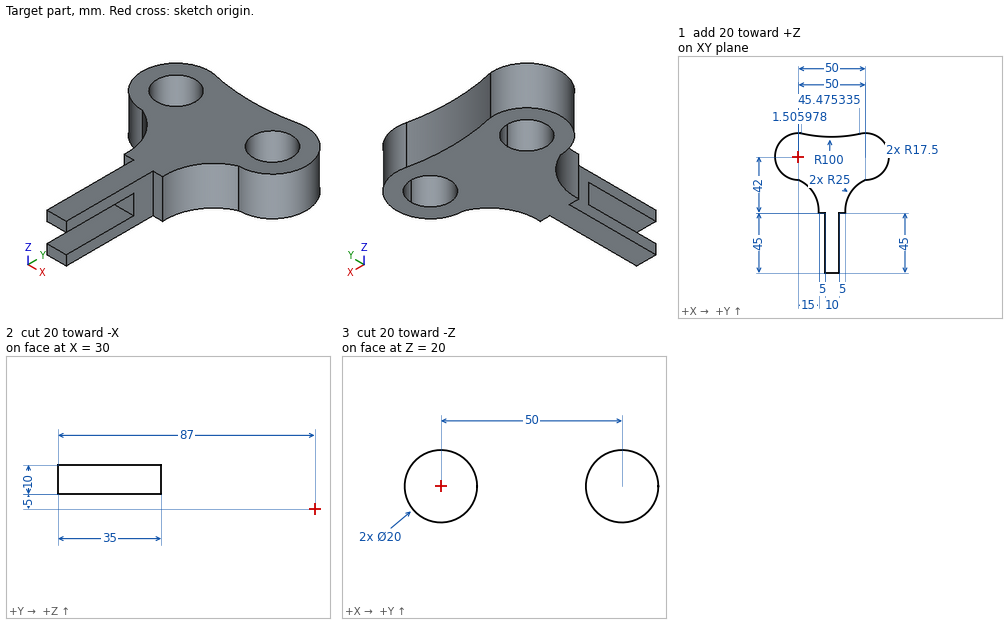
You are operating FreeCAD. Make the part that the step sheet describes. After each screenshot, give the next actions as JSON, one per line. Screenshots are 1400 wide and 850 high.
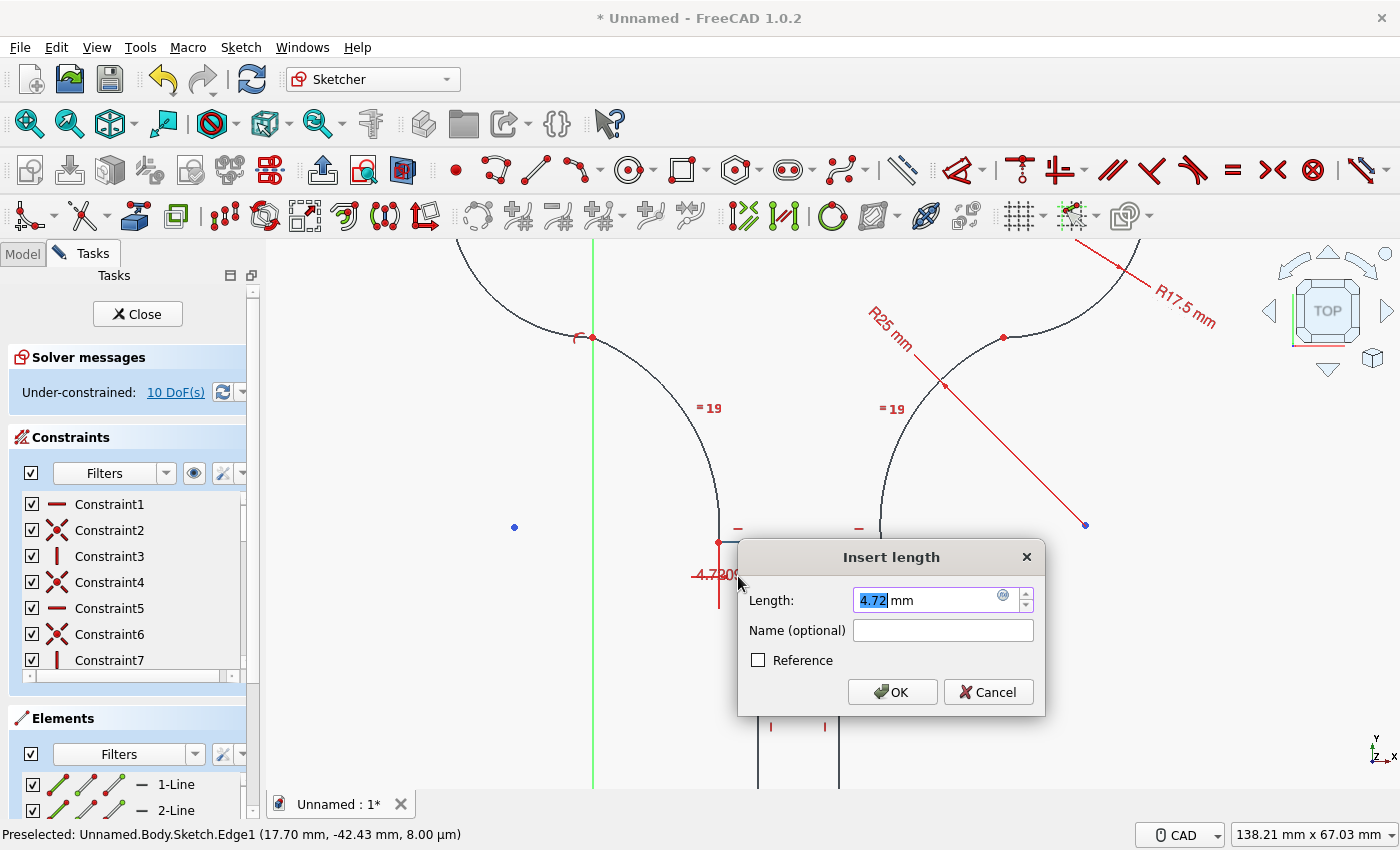
{"action": "type", "text": "5"}
{"action": "key", "text": "Return"}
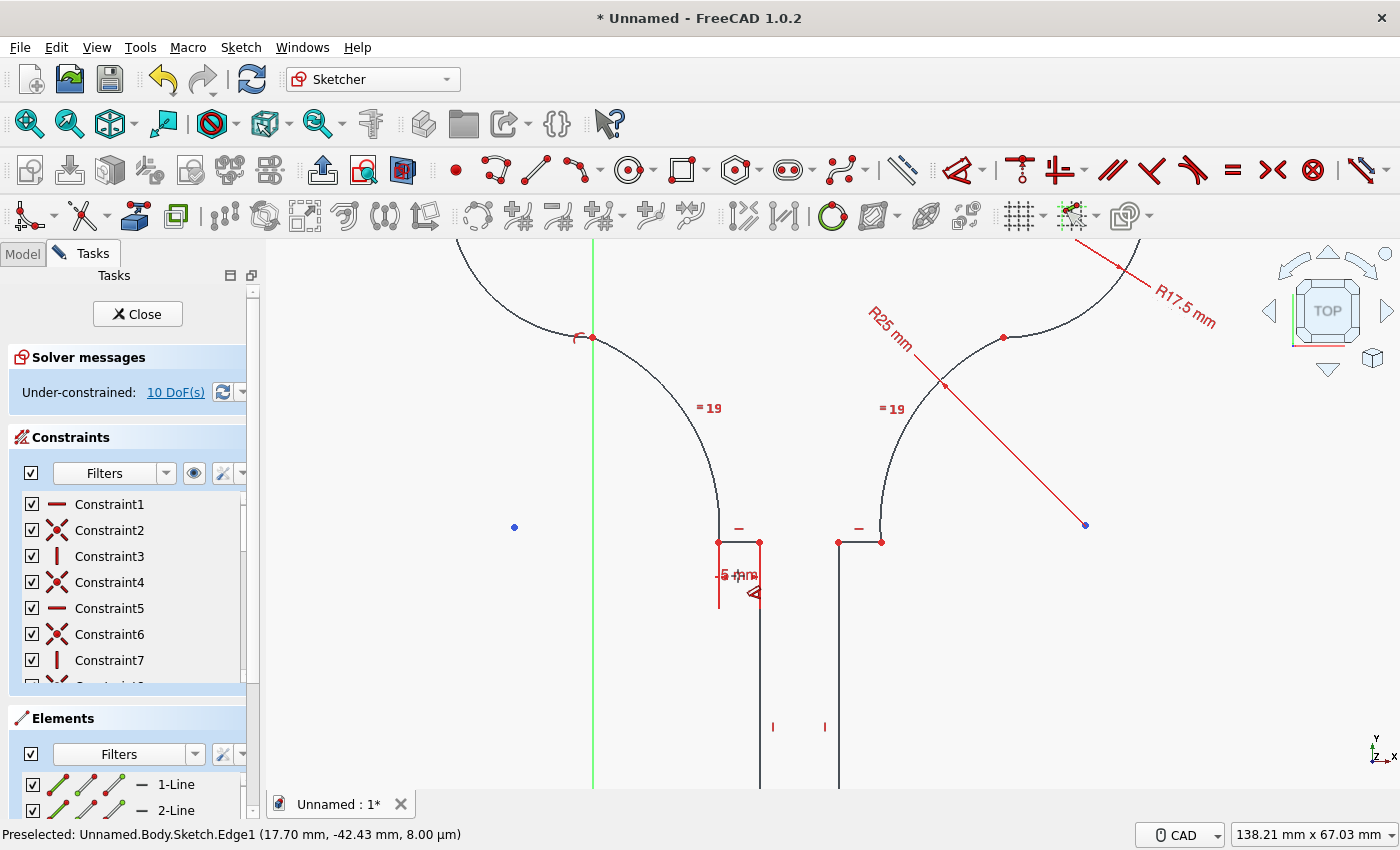
{"action": "left_click", "coordinate": [851, 542]}
{"action": "left_click", "coordinate": [860, 576]}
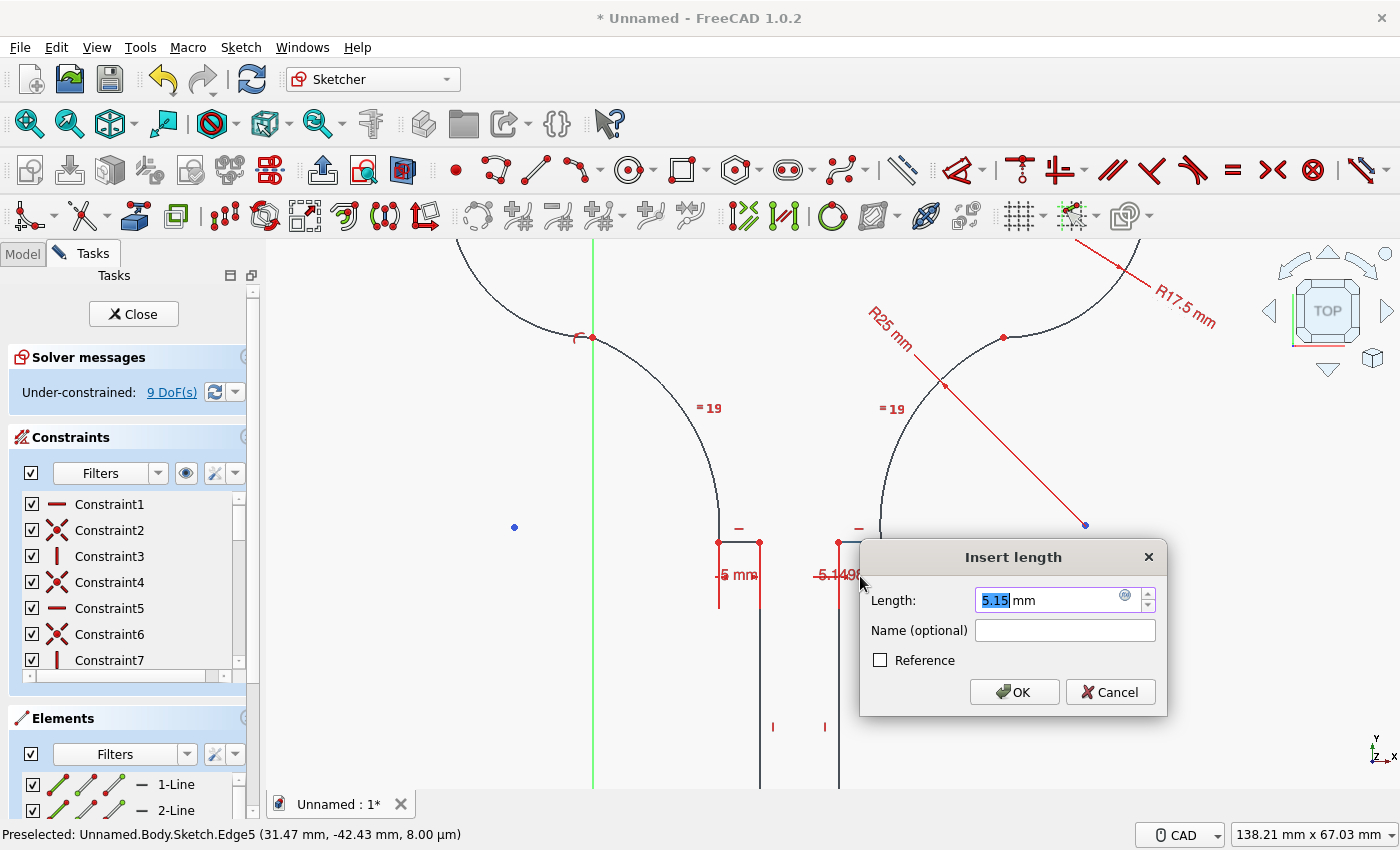
{"action": "type", "text": "5"}
{"action": "key", "text": "Return"}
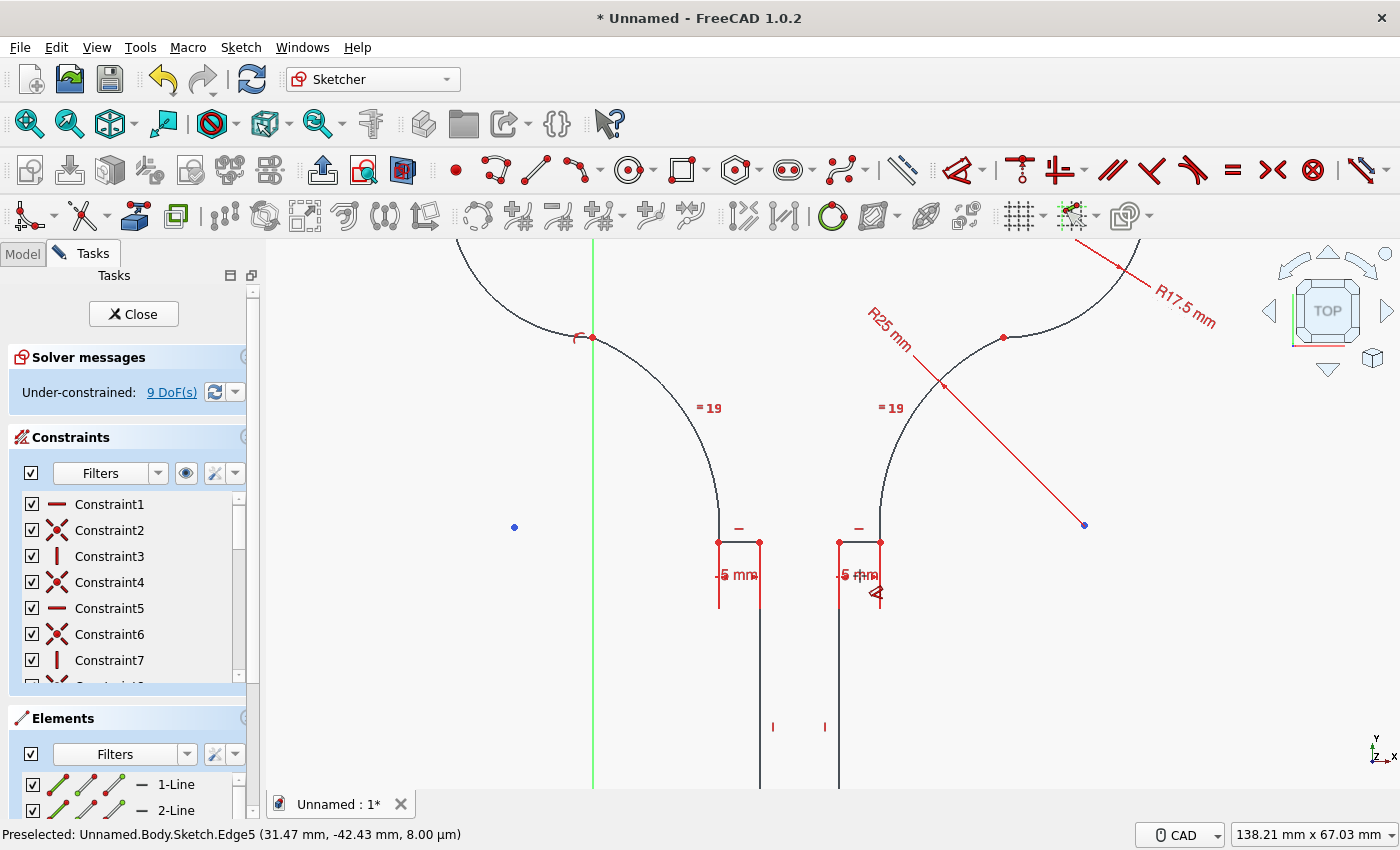
{"action": "left_click", "coordinate": [760, 653]}
{"action": "left_click", "coordinate": [726, 652]}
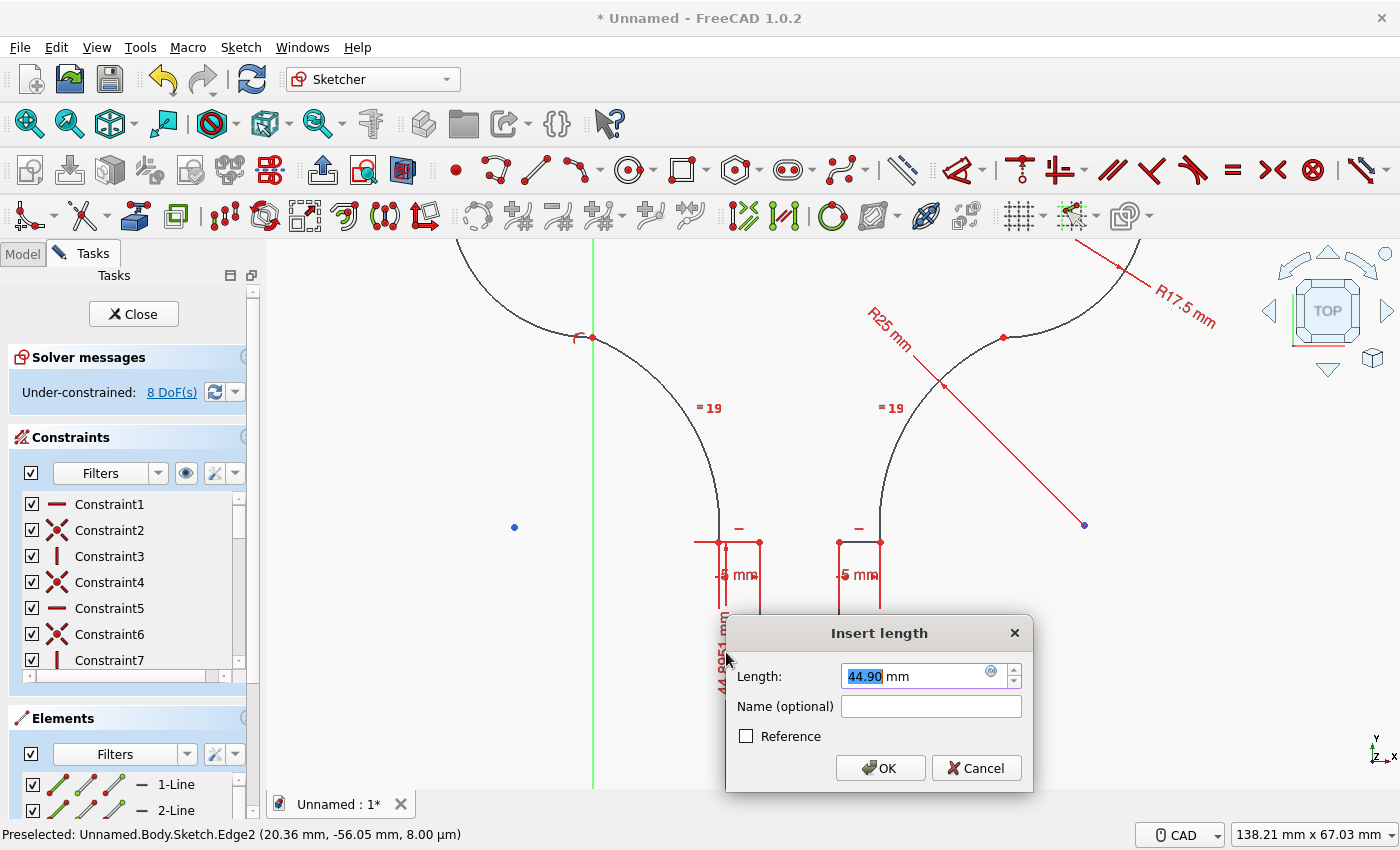
{"action": "type", "text": "45"}
{"action": "key", "text": "Return"}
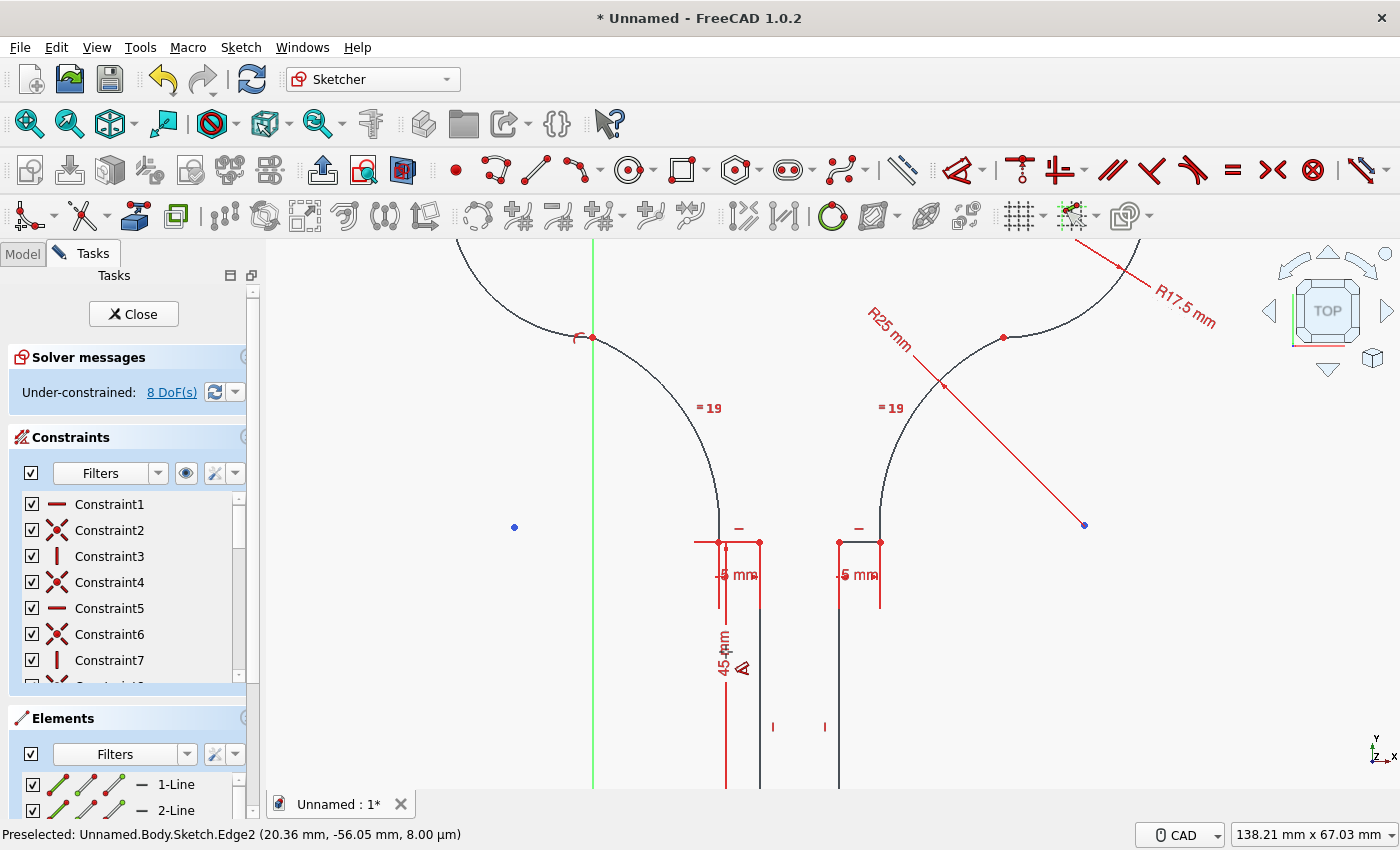
{"action": "scroll", "coordinate": [738, 542], "scroll_direction": "down", "scroll_amount": 4}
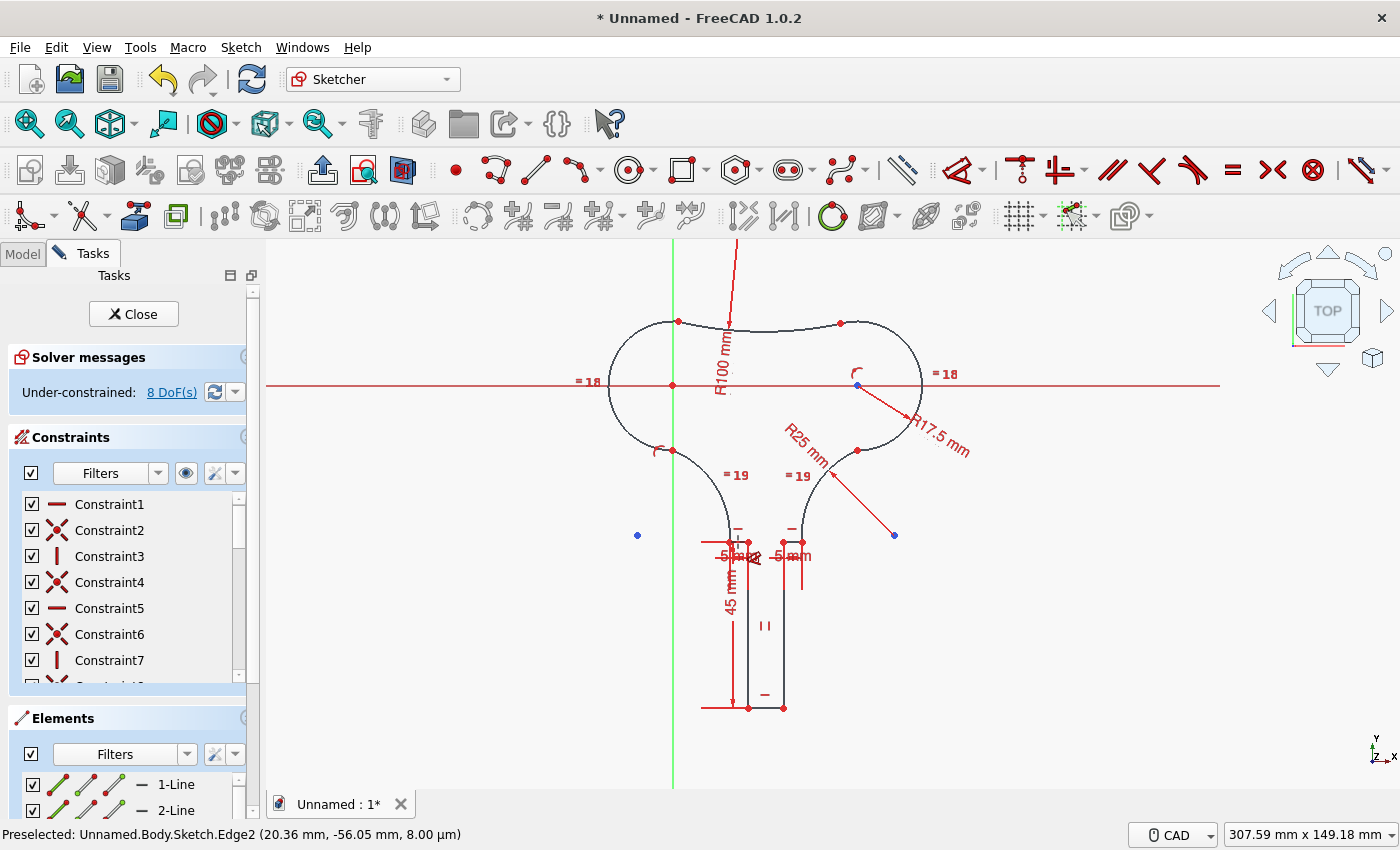
{"action": "scroll", "coordinate": [759, 708], "scroll_direction": "up", "scroll_amount": 2}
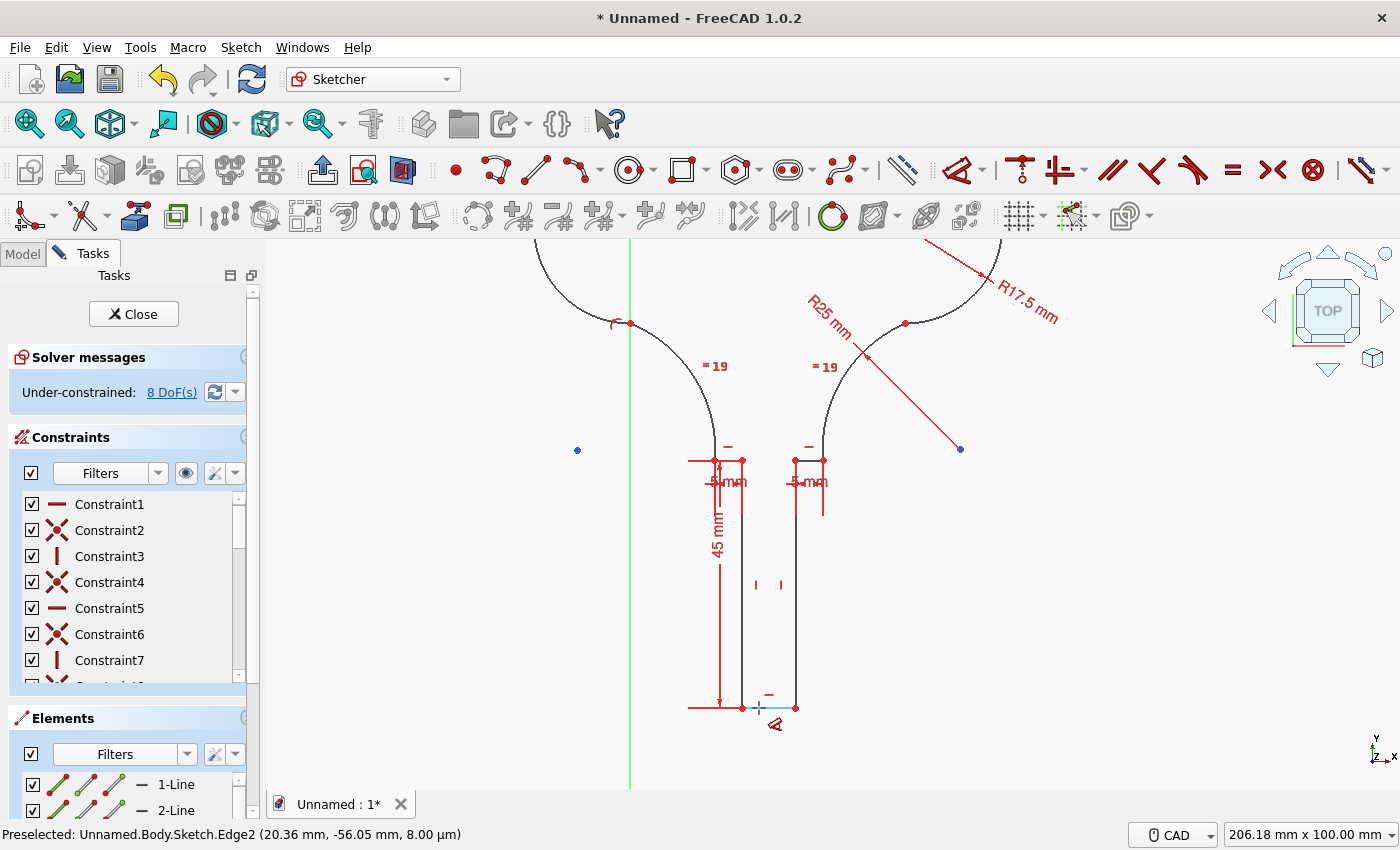
{"action": "left_click", "coordinate": [758, 708]}
{"action": "left_click", "coordinate": [769, 742]}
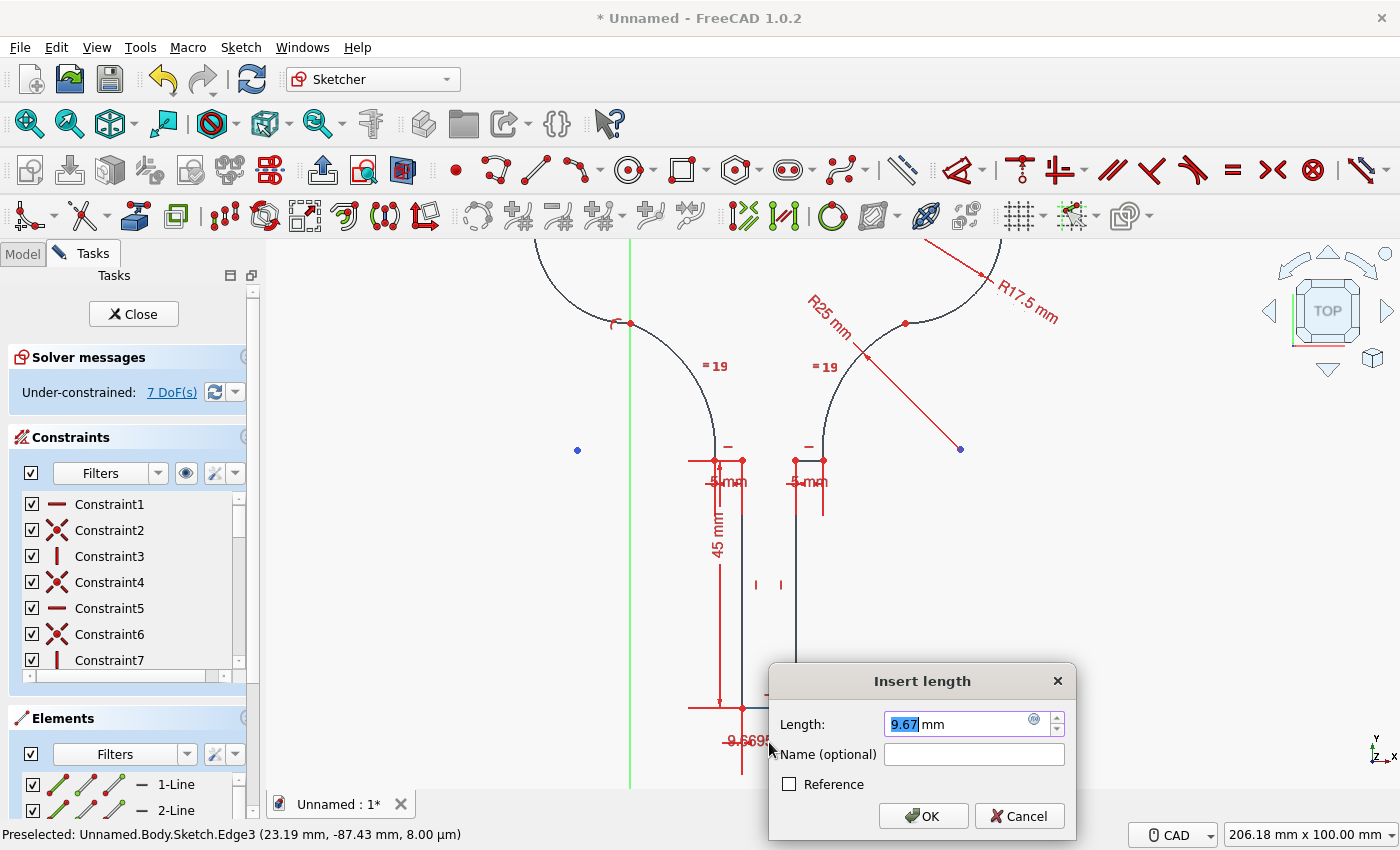
{"action": "type", "text": "10"}
{"action": "key", "text": "Return"}